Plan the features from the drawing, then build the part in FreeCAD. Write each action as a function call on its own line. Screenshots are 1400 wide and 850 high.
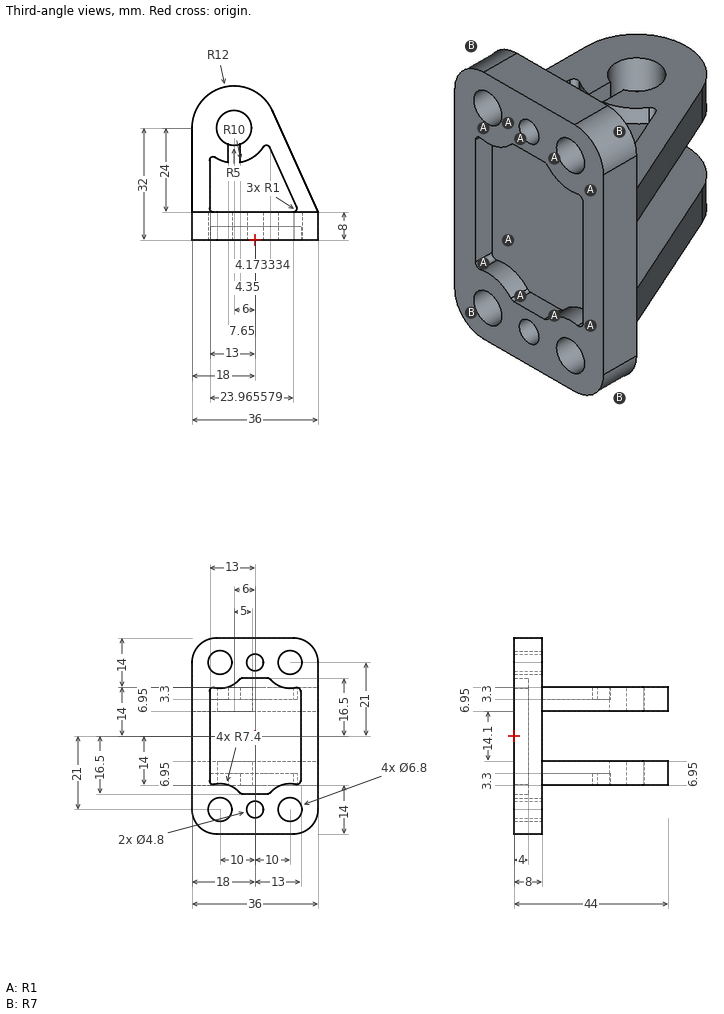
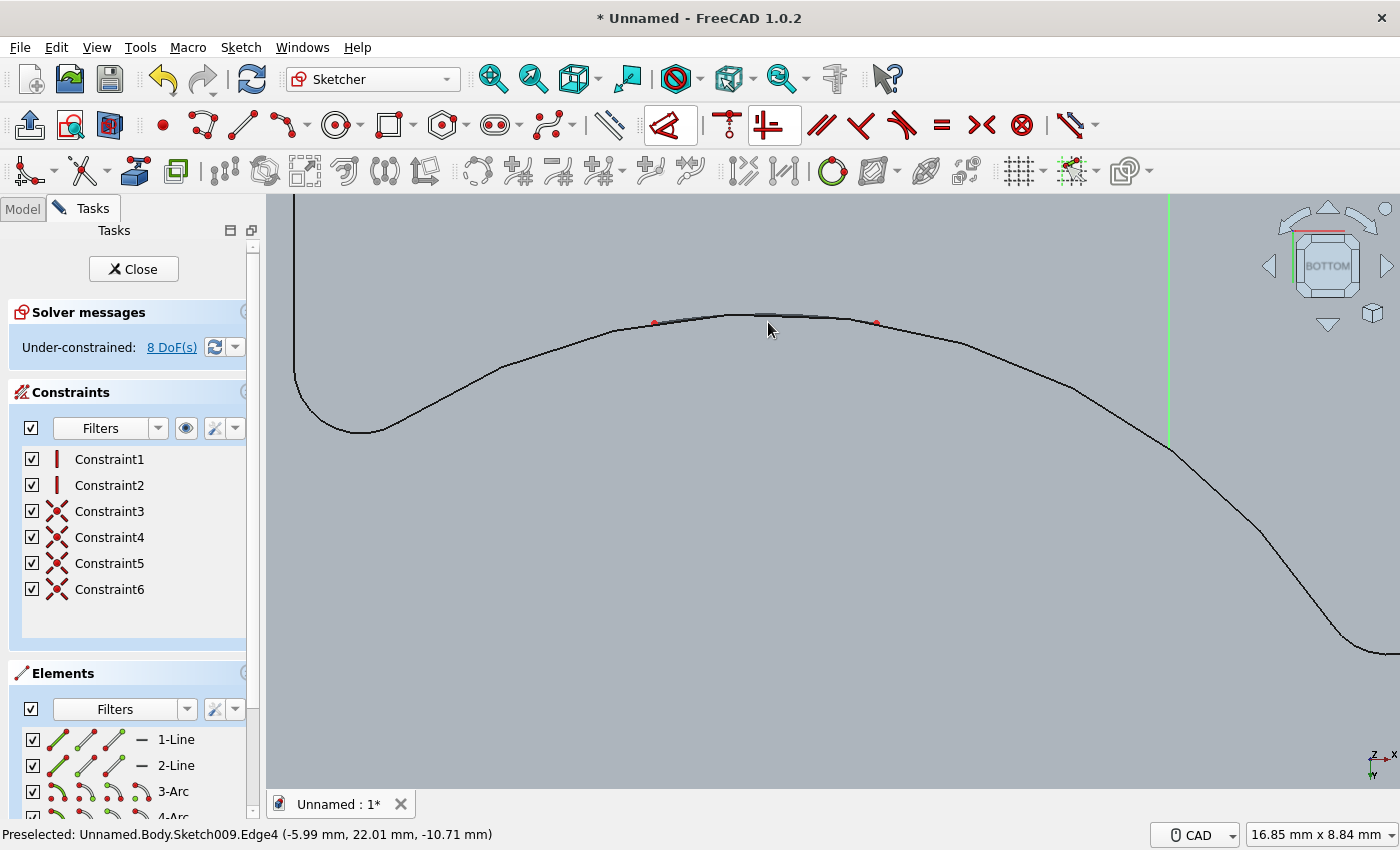
click(810, 654)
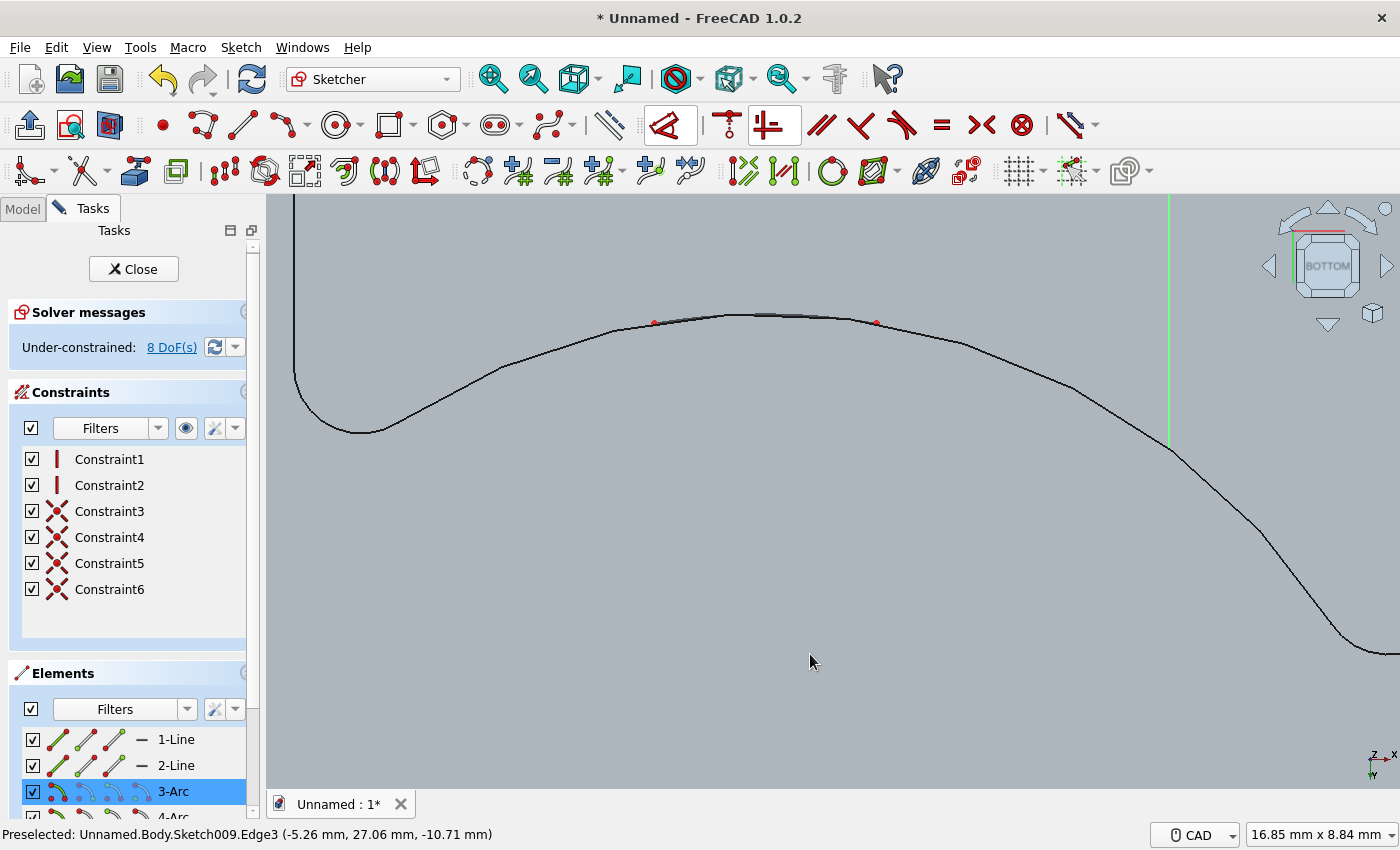
click(810, 316)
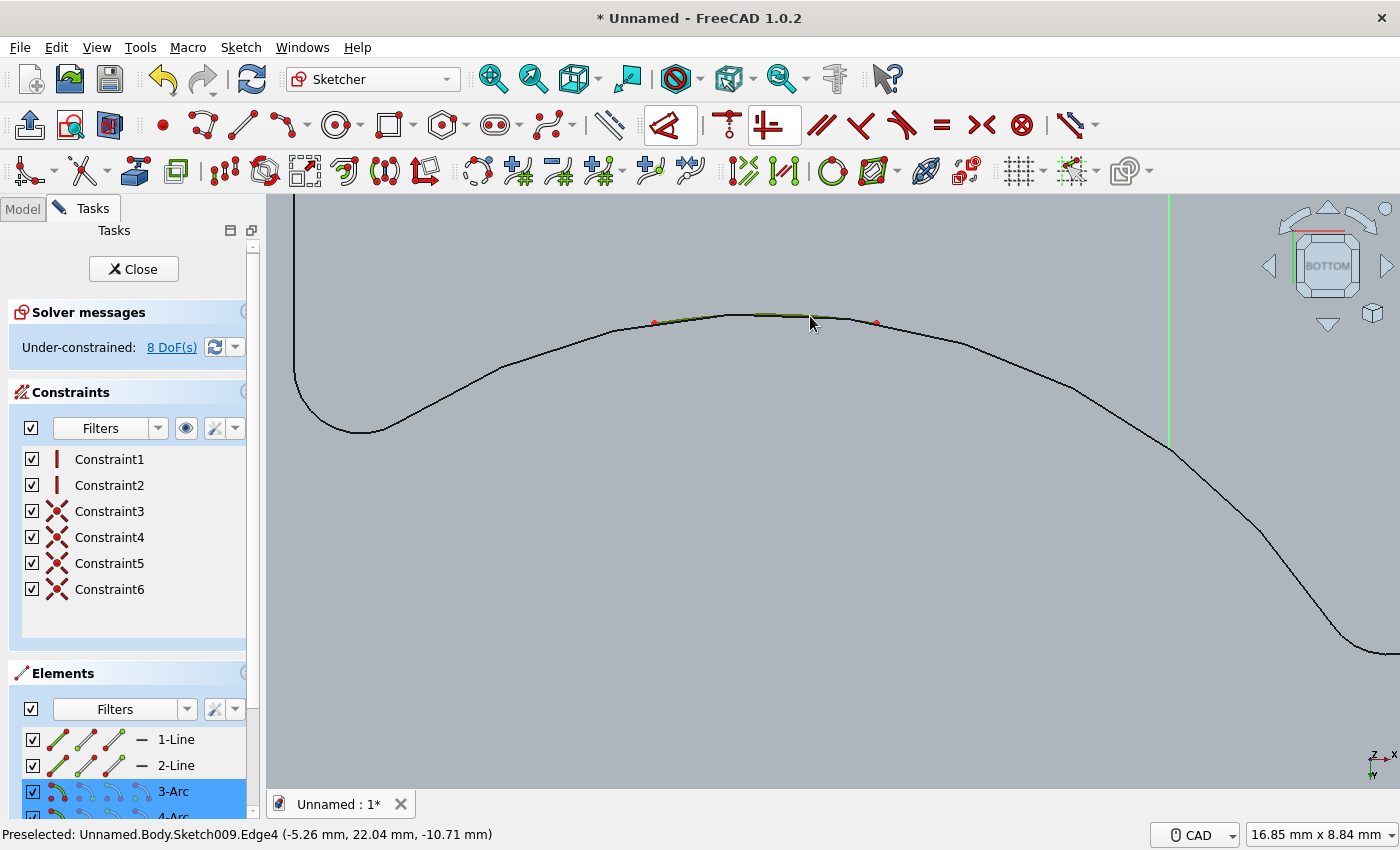
key(c)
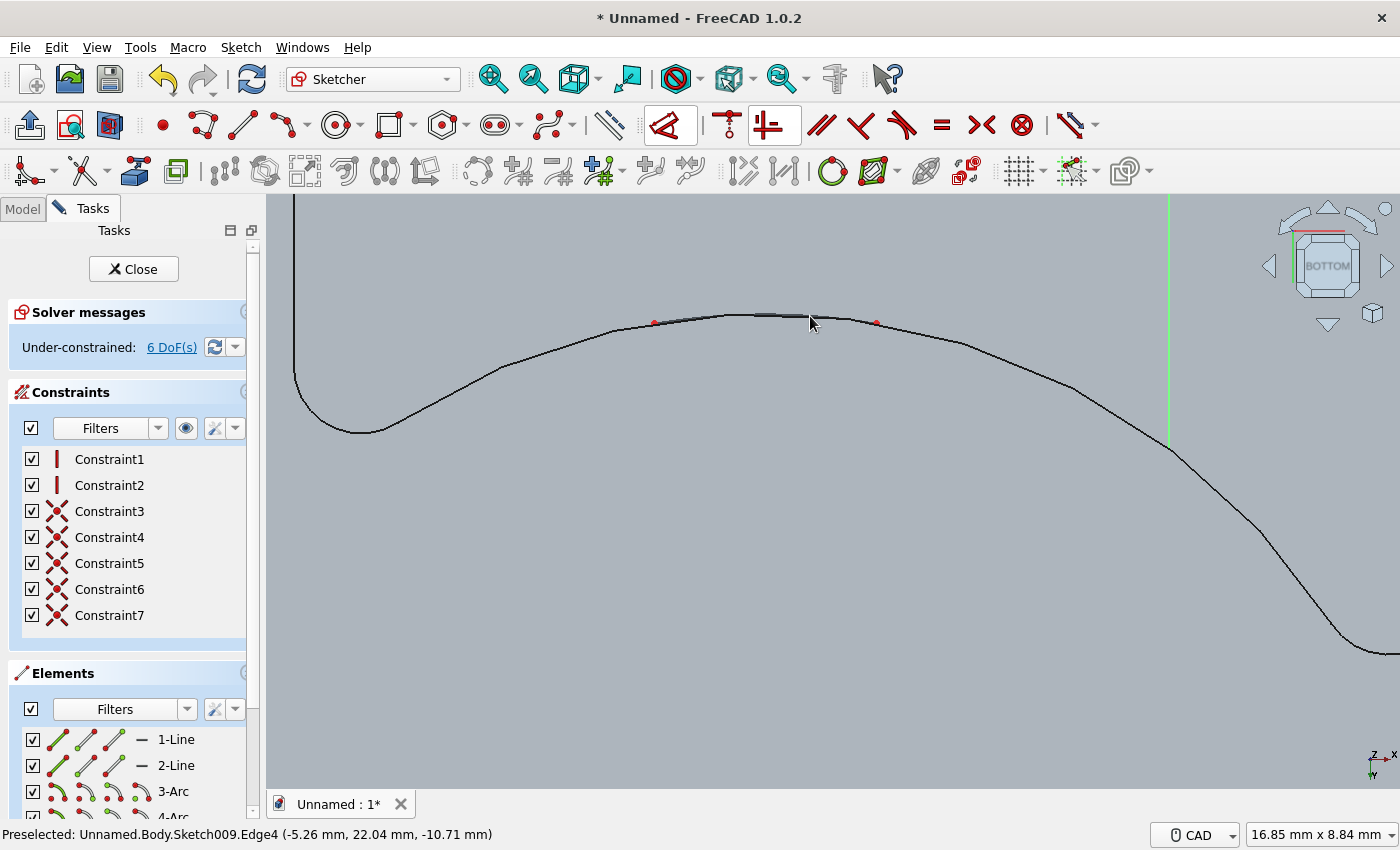
click(810, 653)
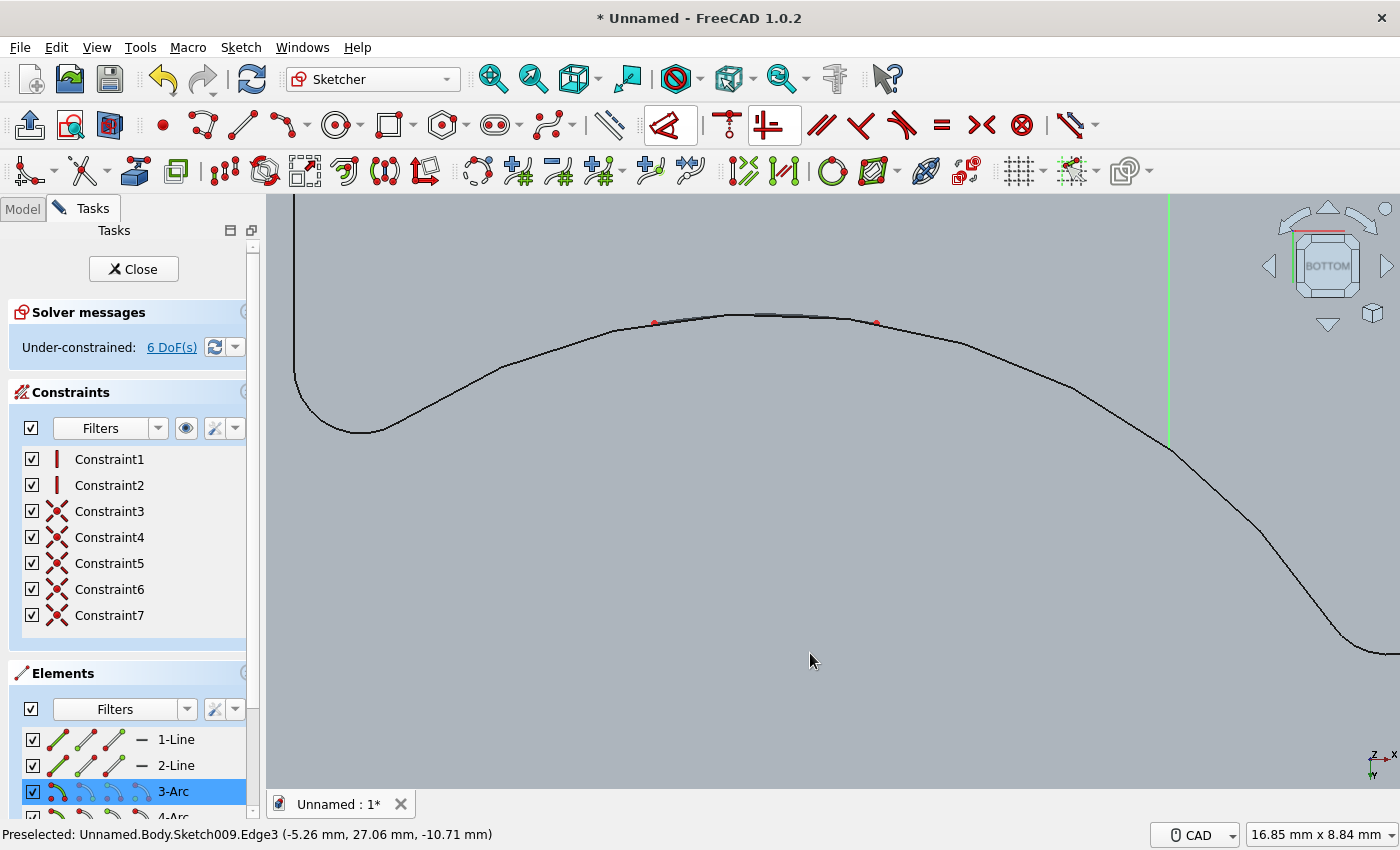
key(k)
key(r)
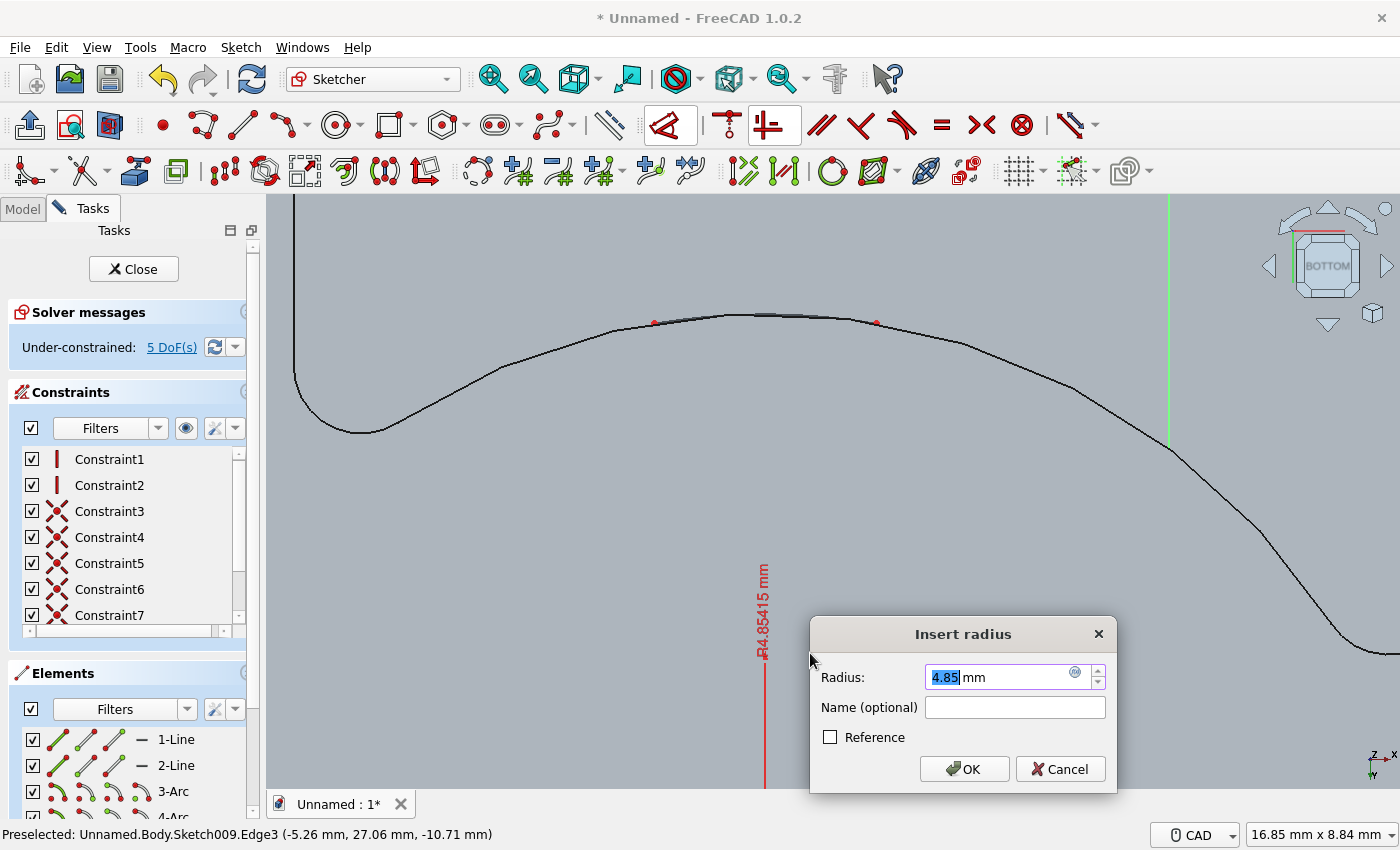
text(5)
key(Return)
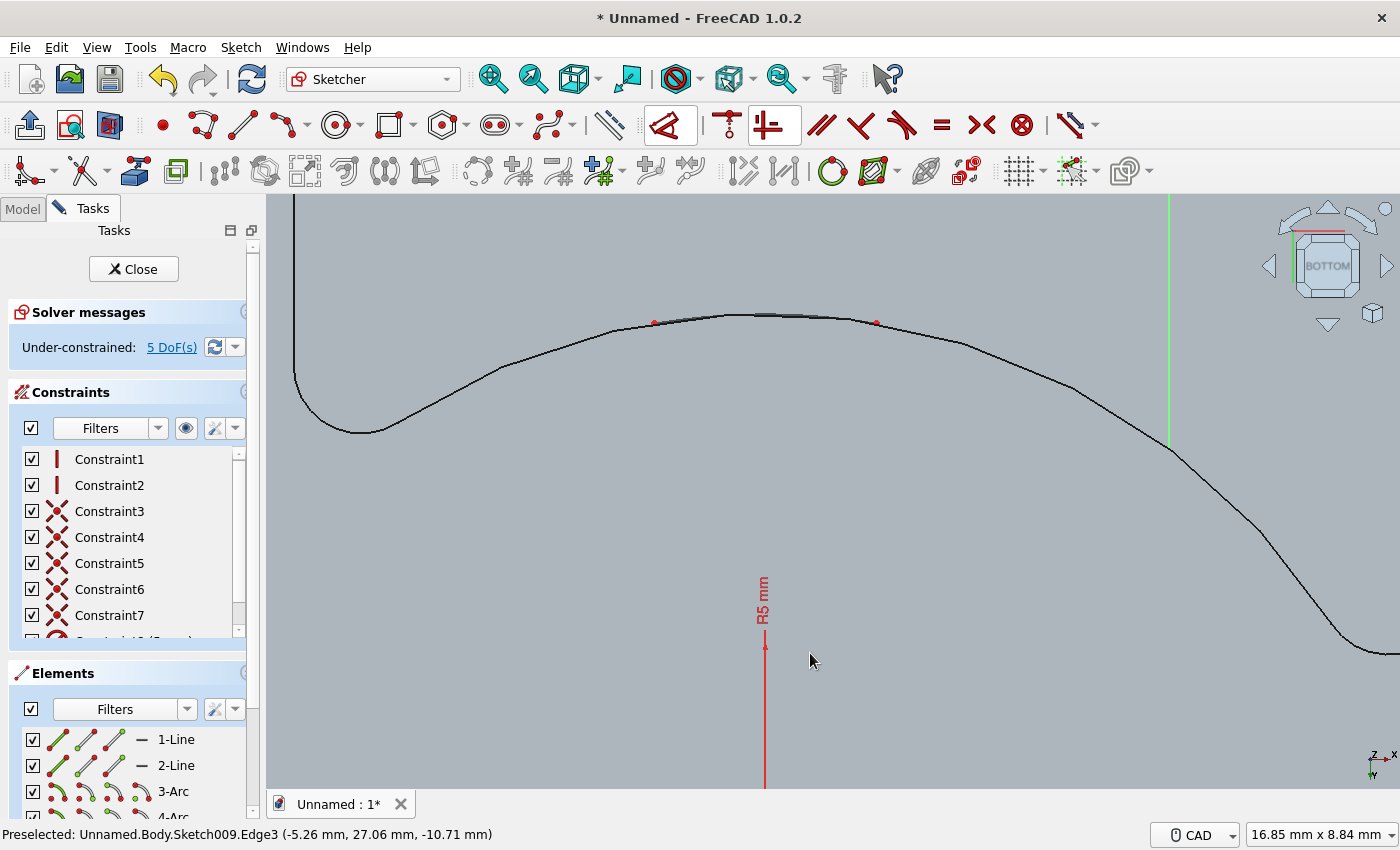
click(810, 316)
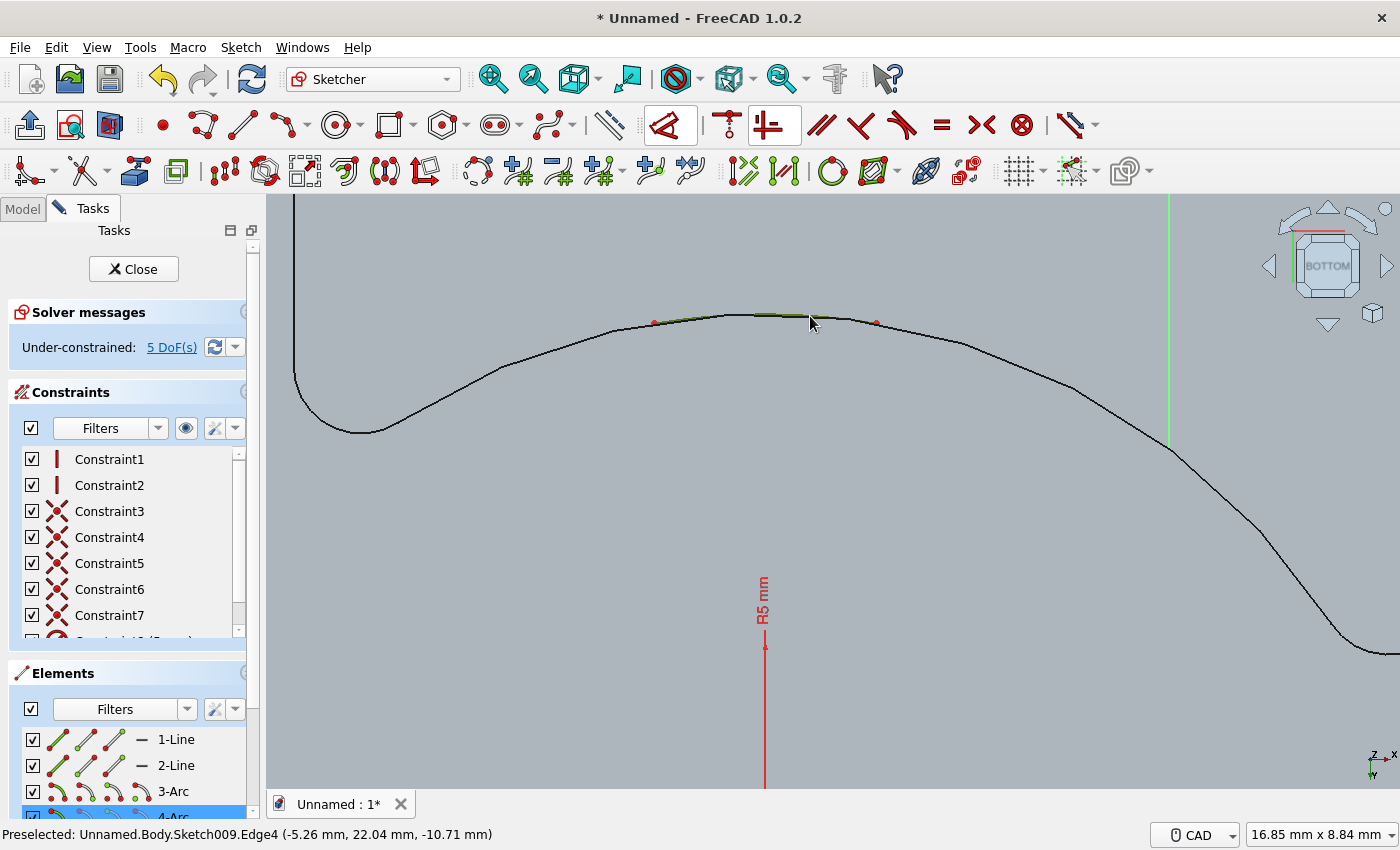
key(k)
key(r)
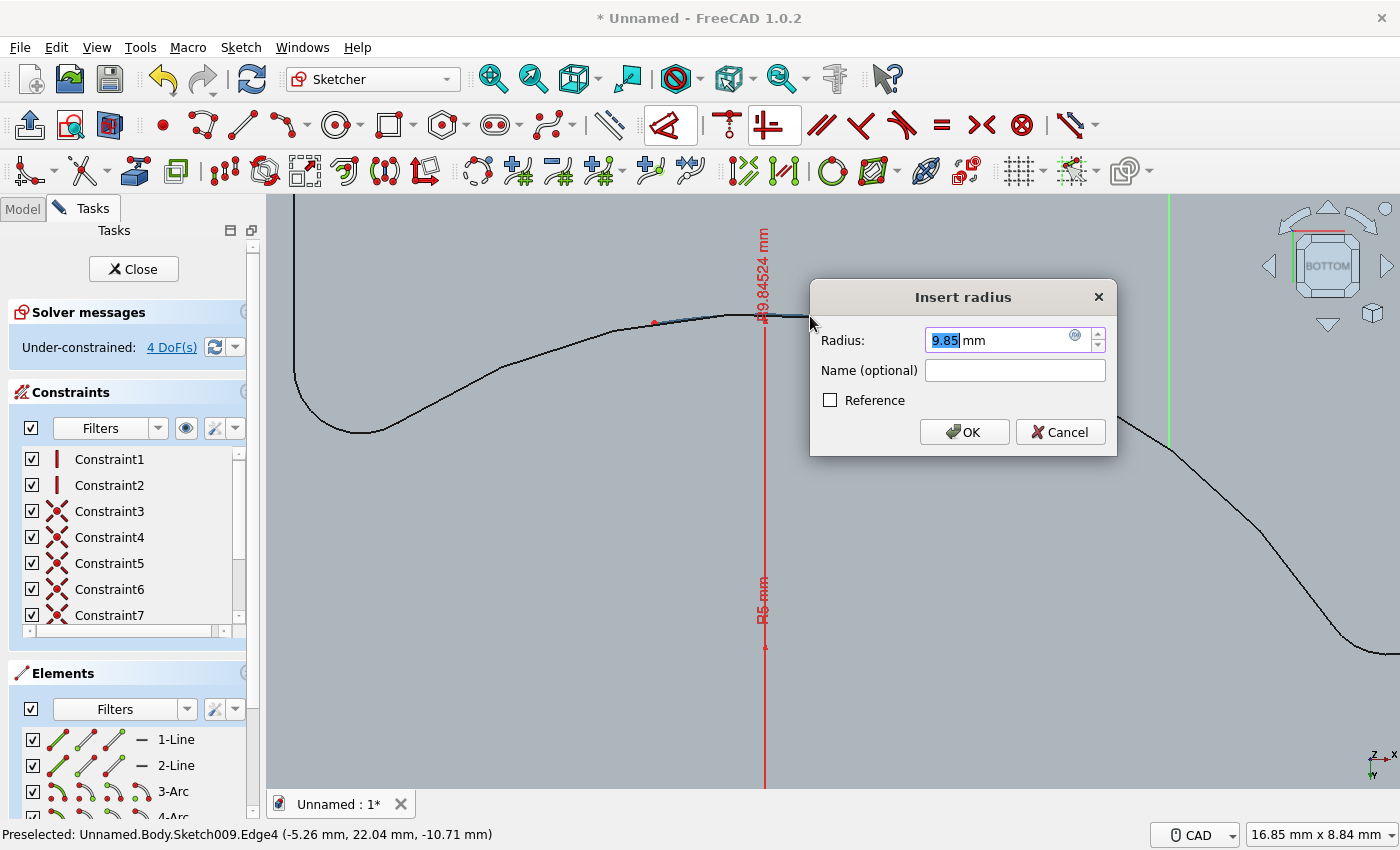
text(10)
key(Return)